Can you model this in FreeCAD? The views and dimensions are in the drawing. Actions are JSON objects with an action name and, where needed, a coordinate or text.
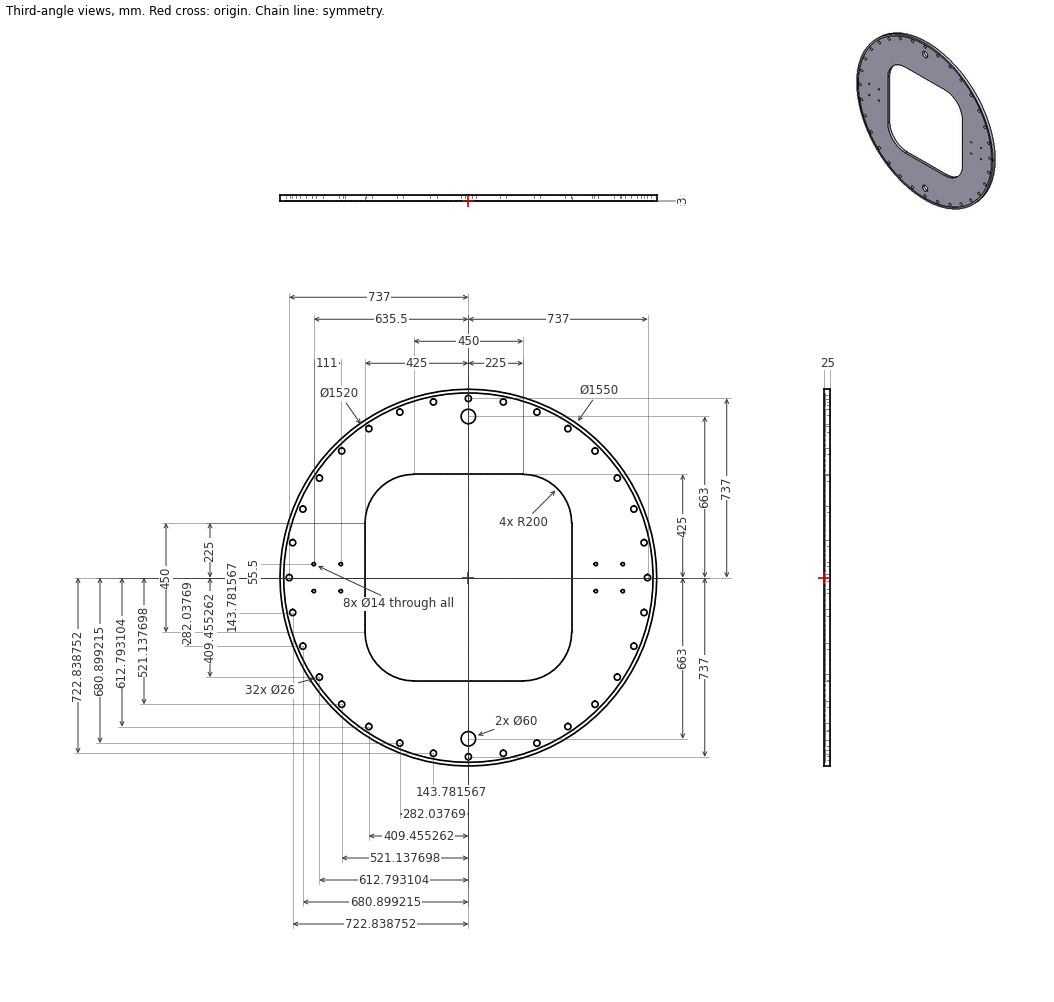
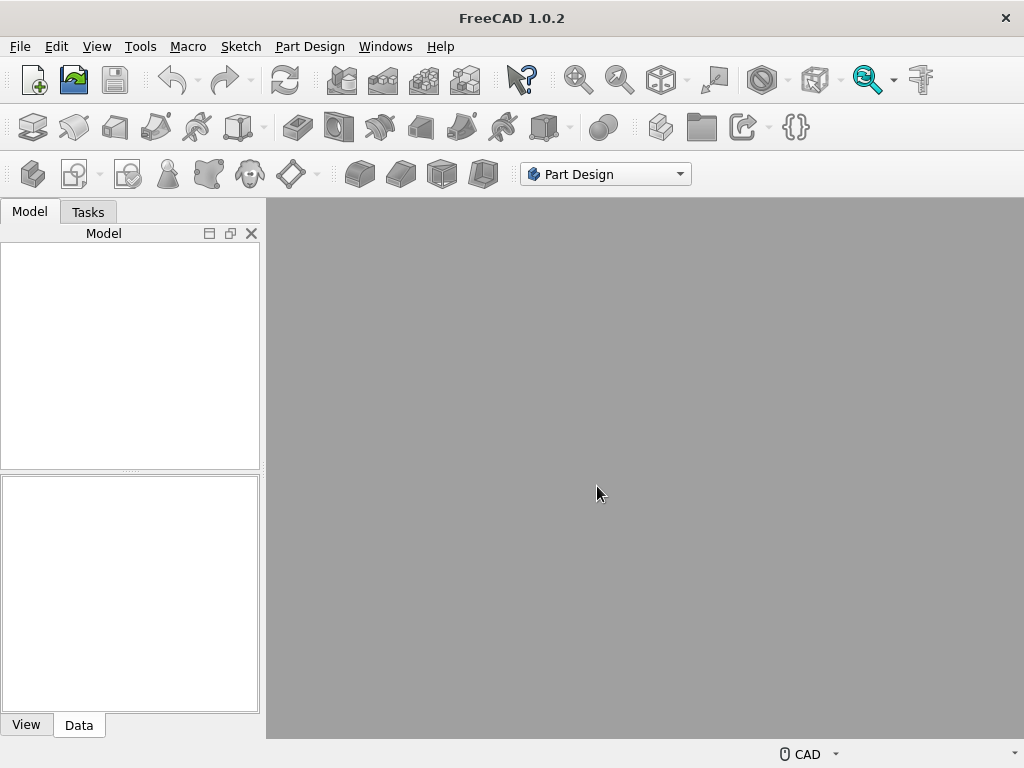
{"action": "left_click", "coordinate": [33, 80]}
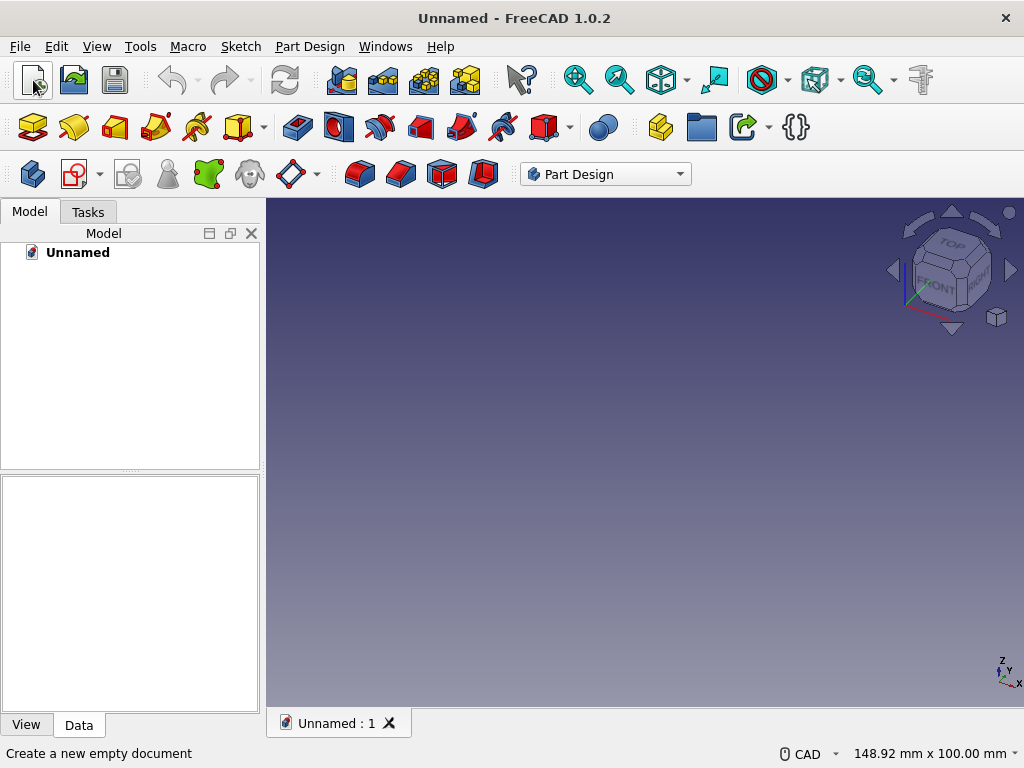
{"action": "left_click", "coordinate": [74, 174]}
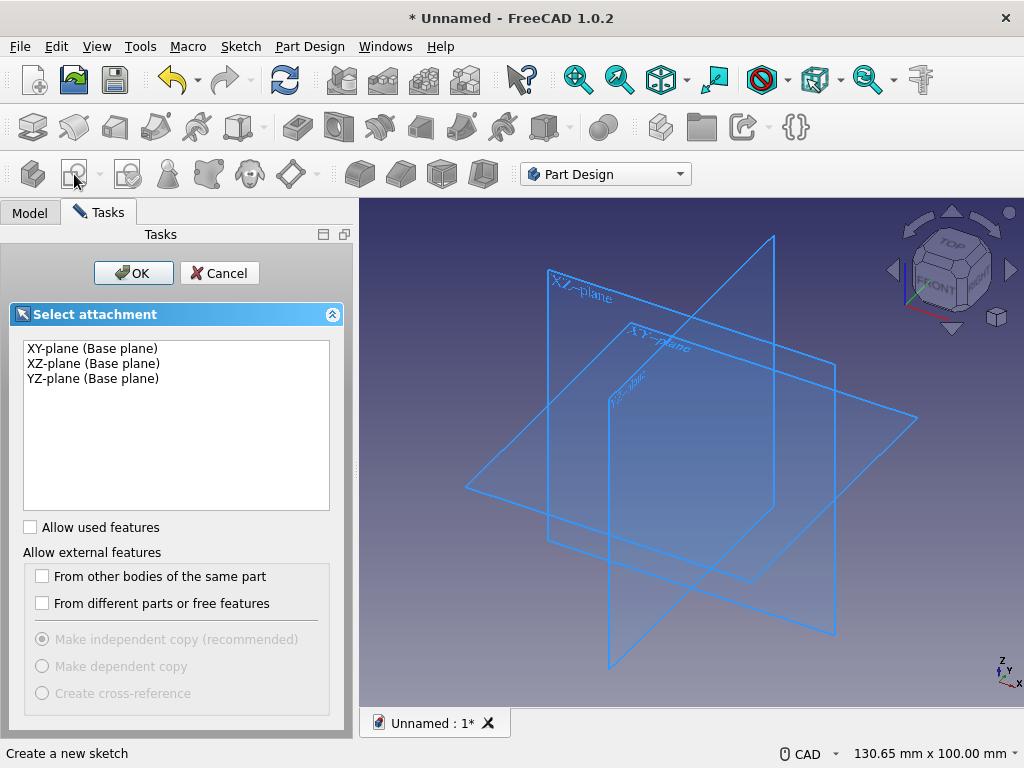
{"action": "left_click", "coordinate": [84, 364]}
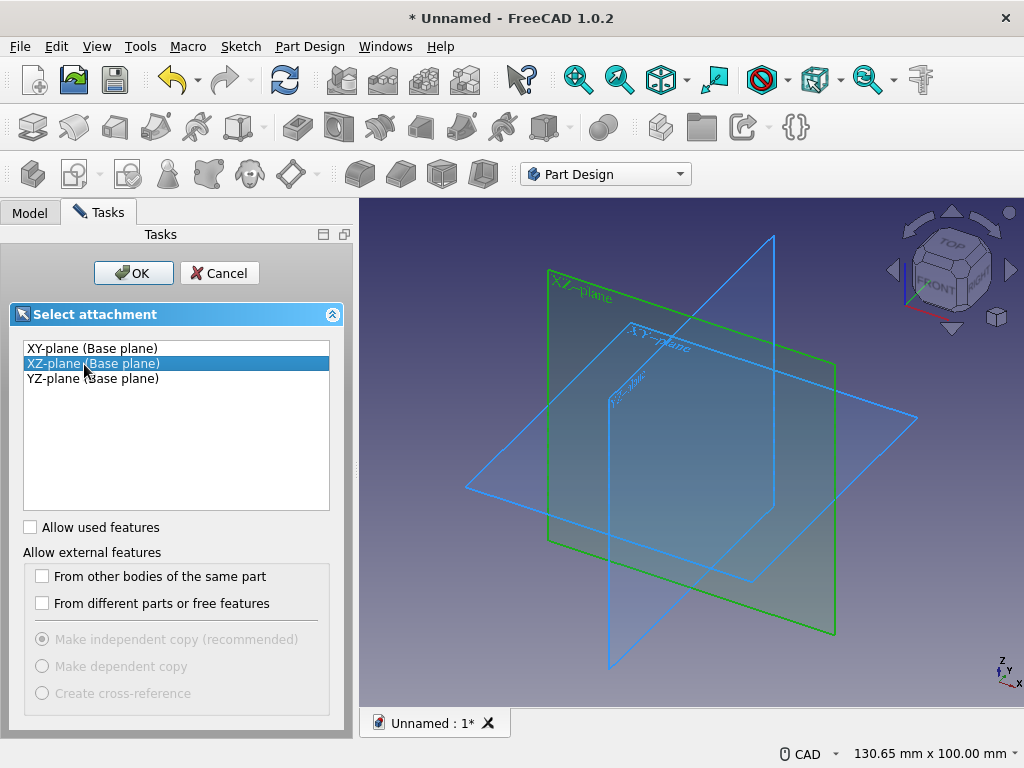
{"action": "left_click", "coordinate": [134, 273]}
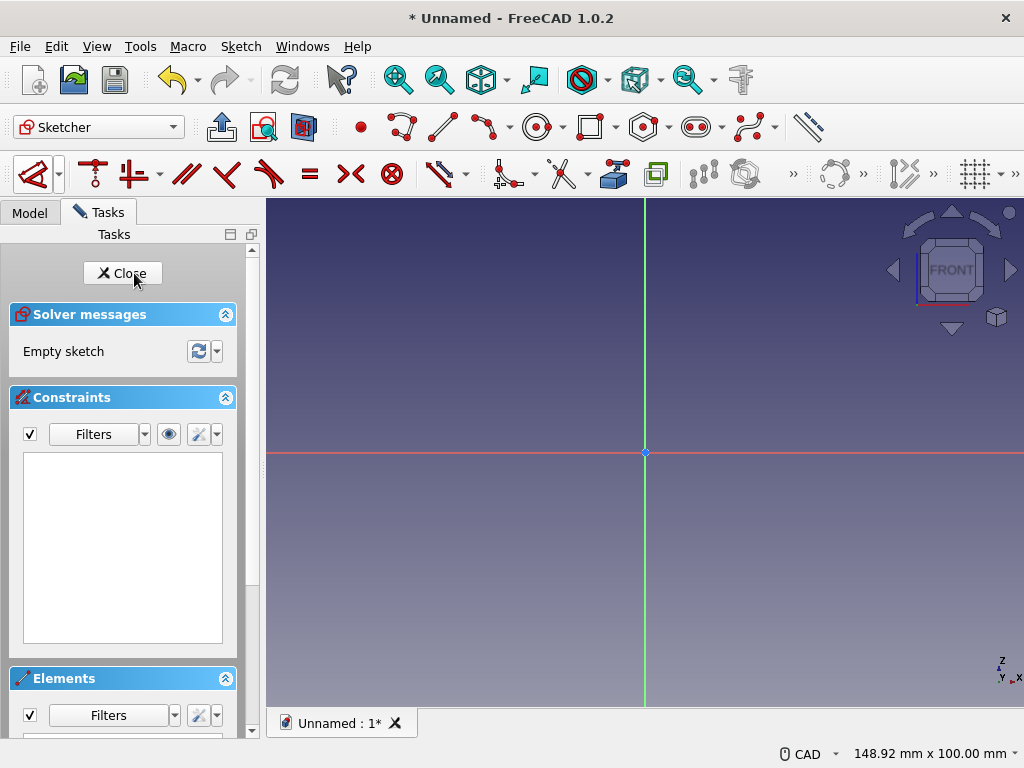
{"action": "scroll", "coordinate": [573, 452], "scroll_direction": "down", "scroll_amount": 15}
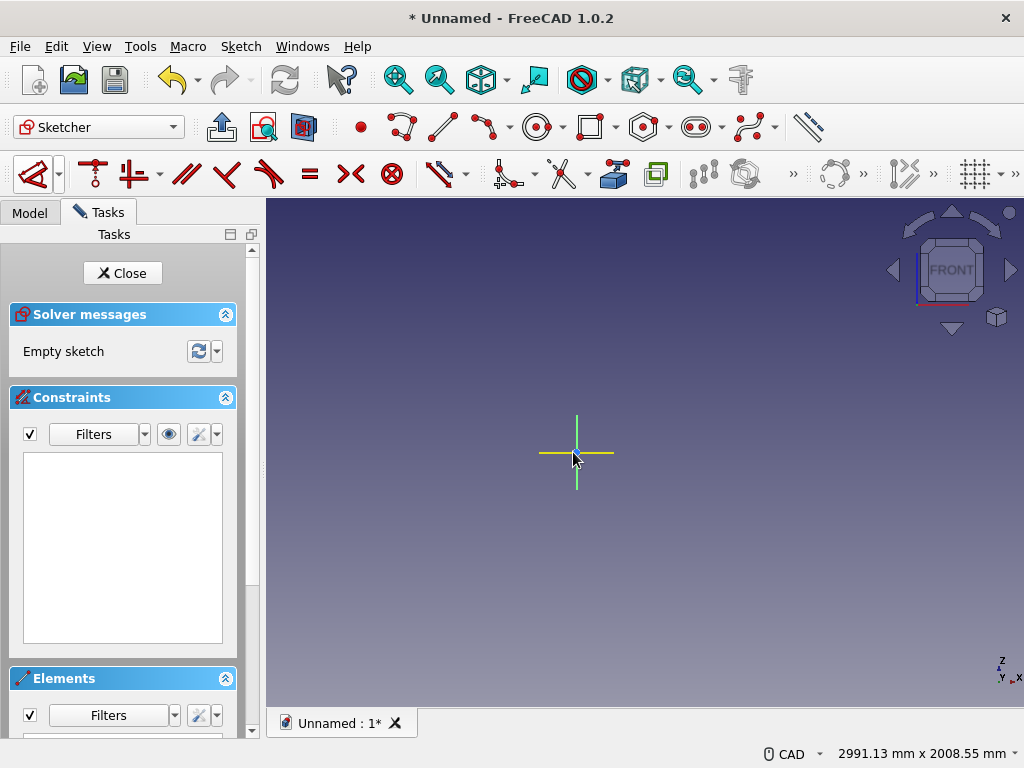
{"action": "left_click", "coordinate": [443, 128]}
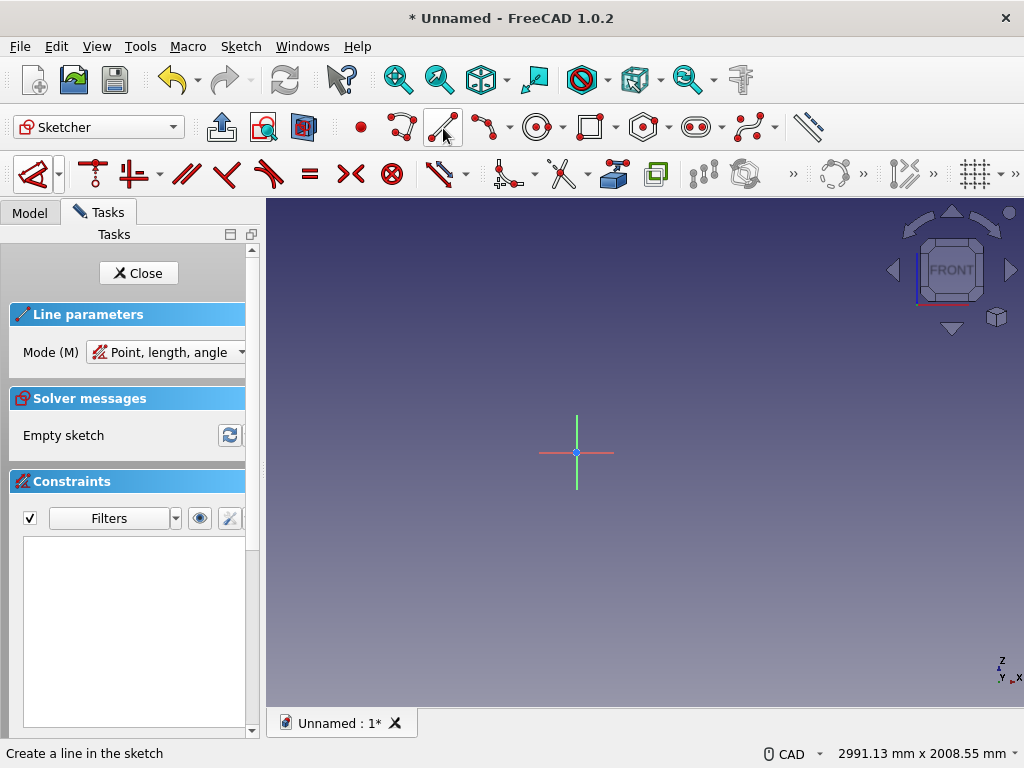
{"action": "left_click", "coordinate": [634, 345]}
{"action": "left_click", "coordinate": [520, 345]}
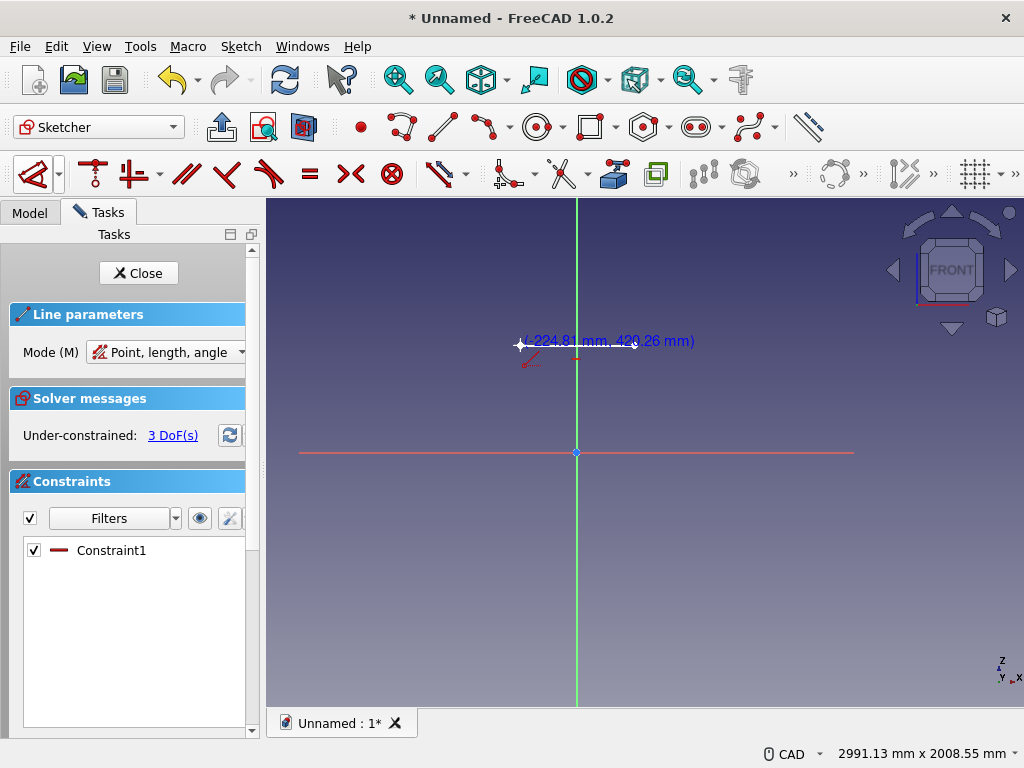
{"action": "left_click", "coordinate": [469, 395]}
{"action": "left_click", "coordinate": [469, 510]}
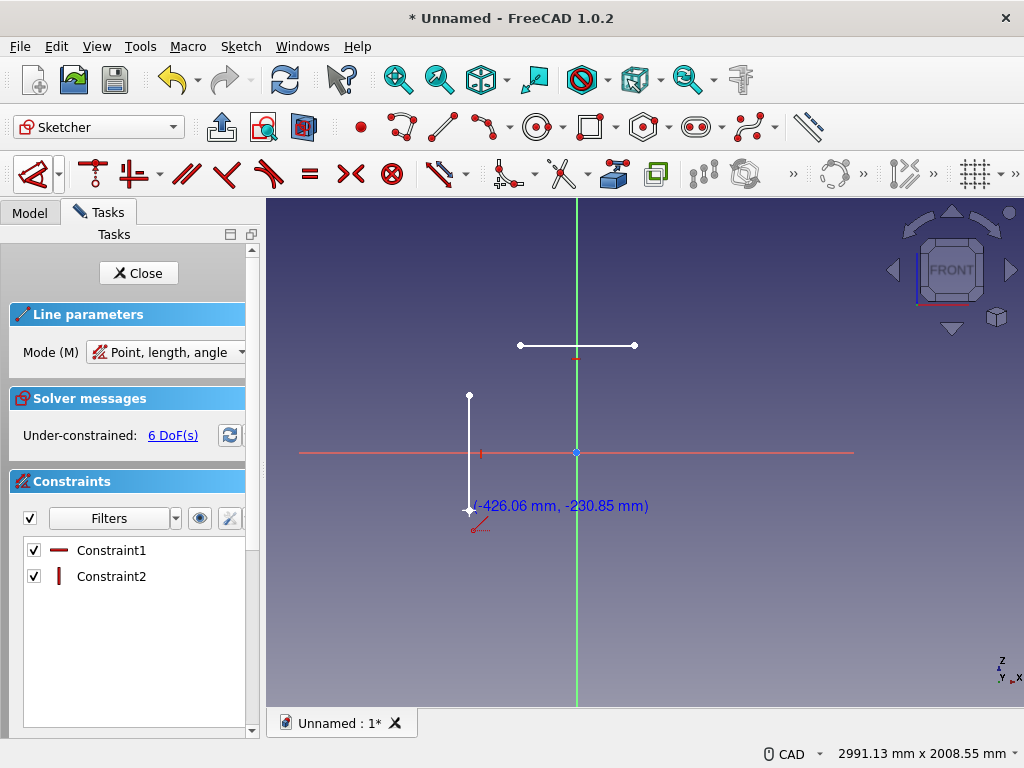
{"action": "left_click", "coordinate": [520, 560]}
{"action": "left_click", "coordinate": [634, 560]}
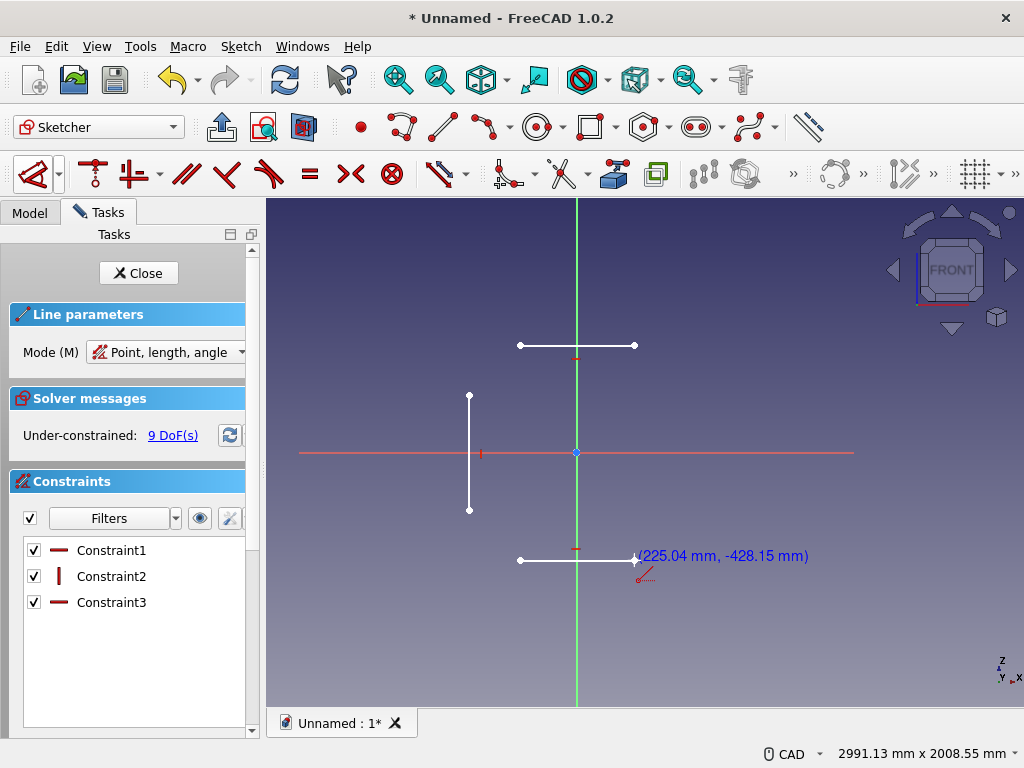
{"action": "left_click", "coordinate": [685, 510]}
{"action": "left_click", "coordinate": [685, 395]}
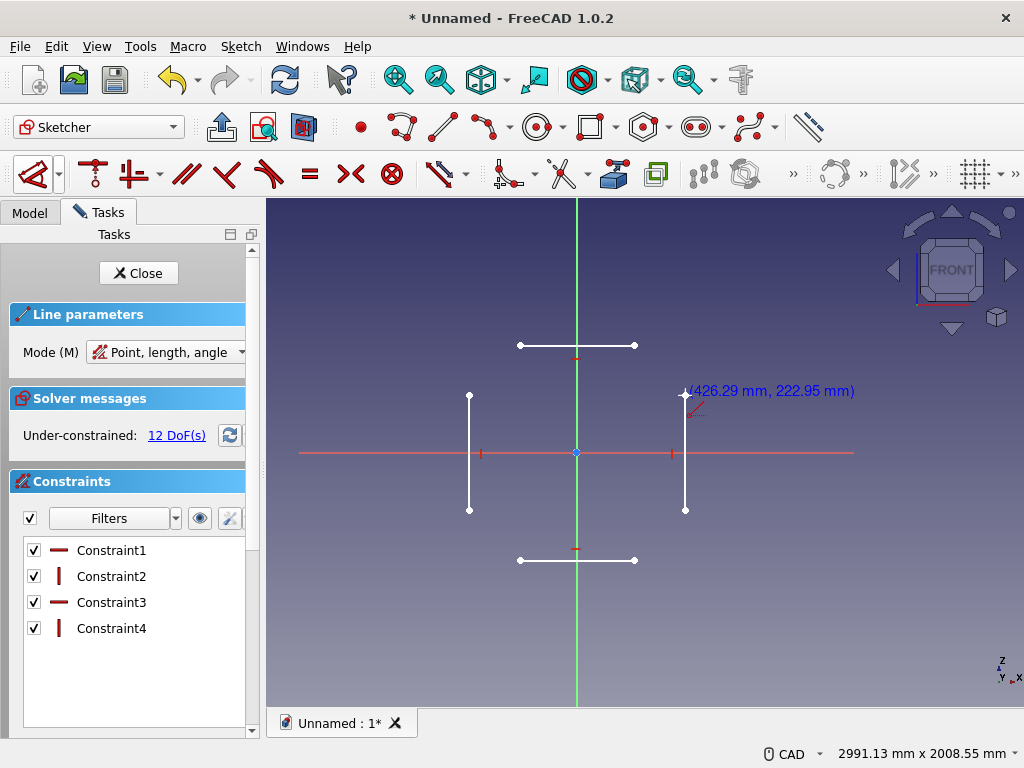
{"action": "left_click", "coordinate": [484, 128]}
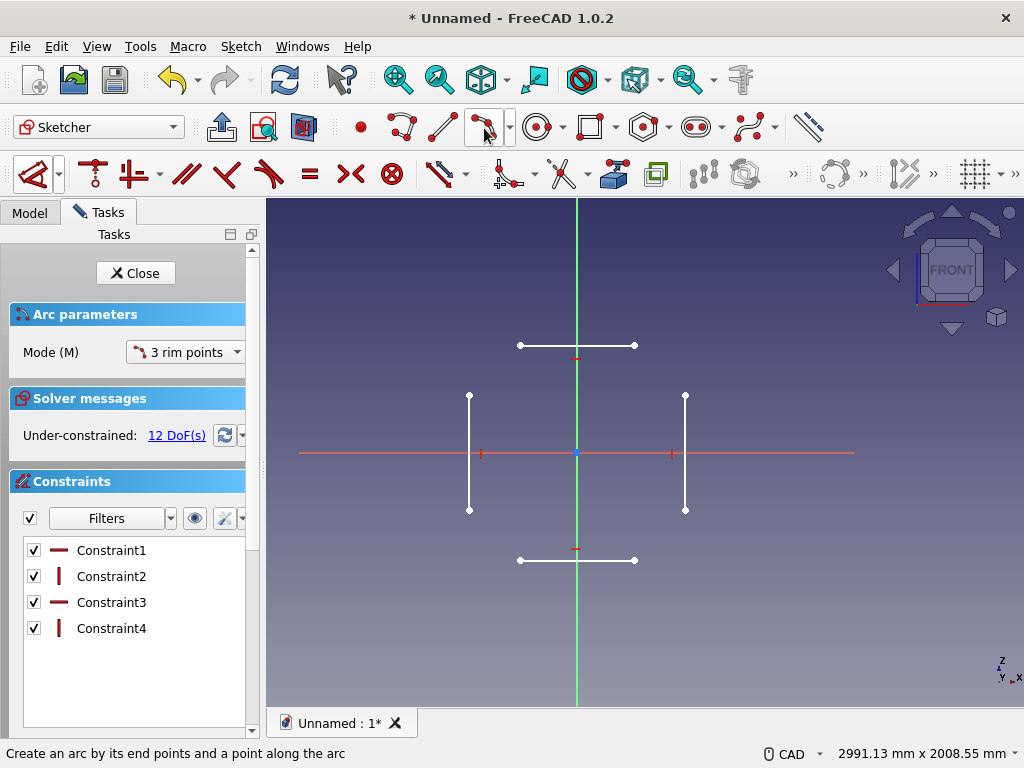
{"action": "left_click", "coordinate": [520, 346]}
{"action": "left_click", "coordinate": [469, 396]}
{"action": "left_click", "coordinate": [484, 360]}